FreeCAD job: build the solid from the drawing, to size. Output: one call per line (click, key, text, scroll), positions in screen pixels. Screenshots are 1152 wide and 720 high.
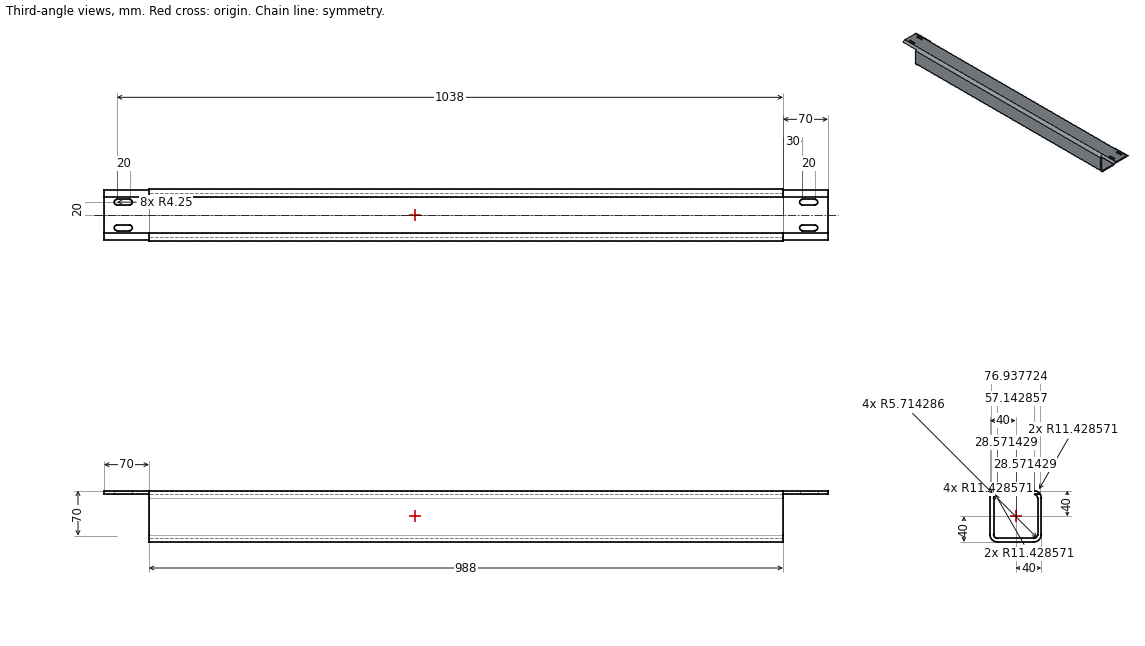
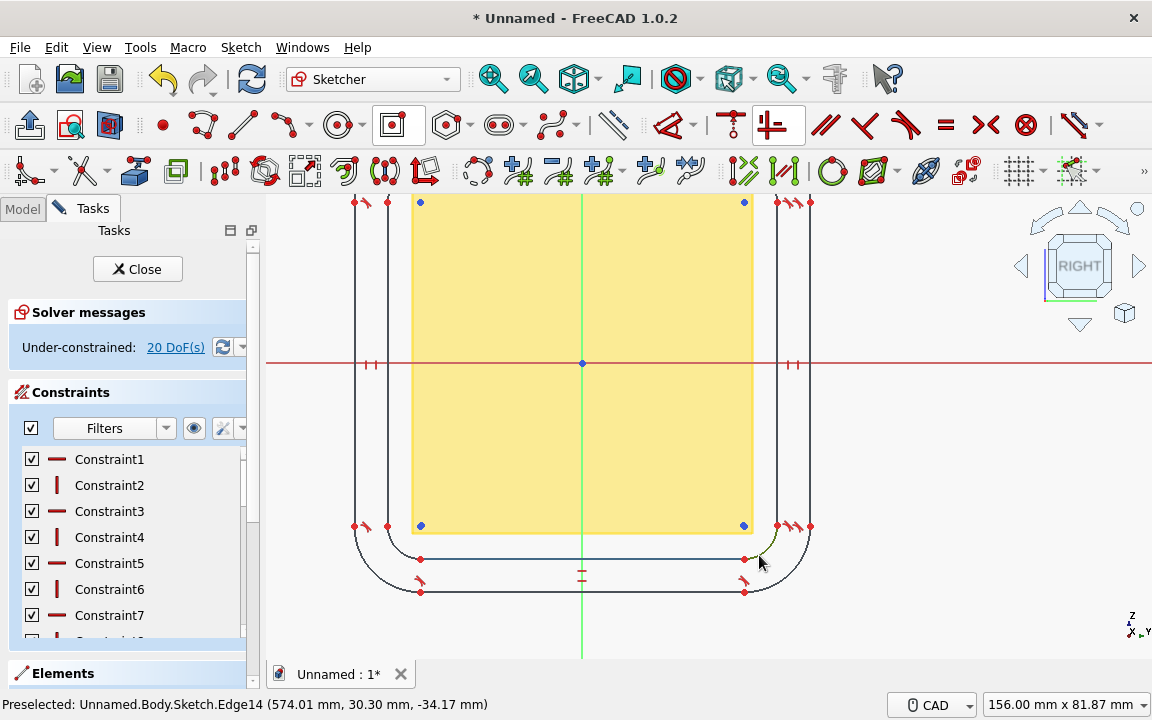
key(t)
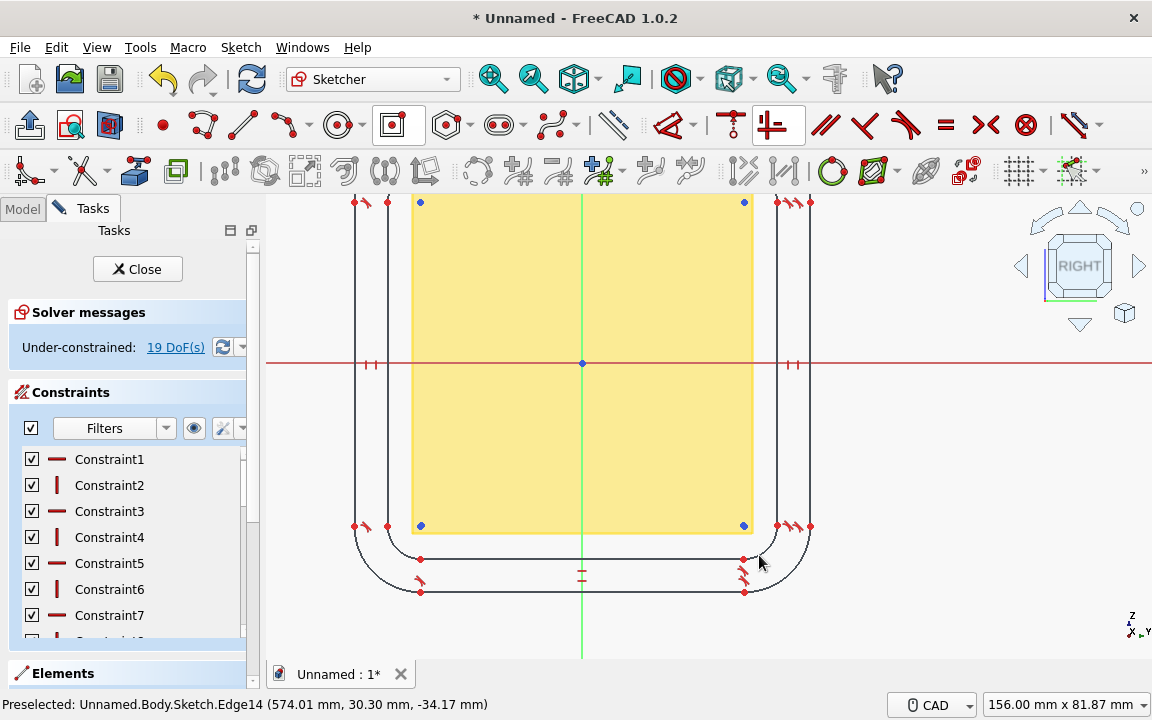
click(647, 559)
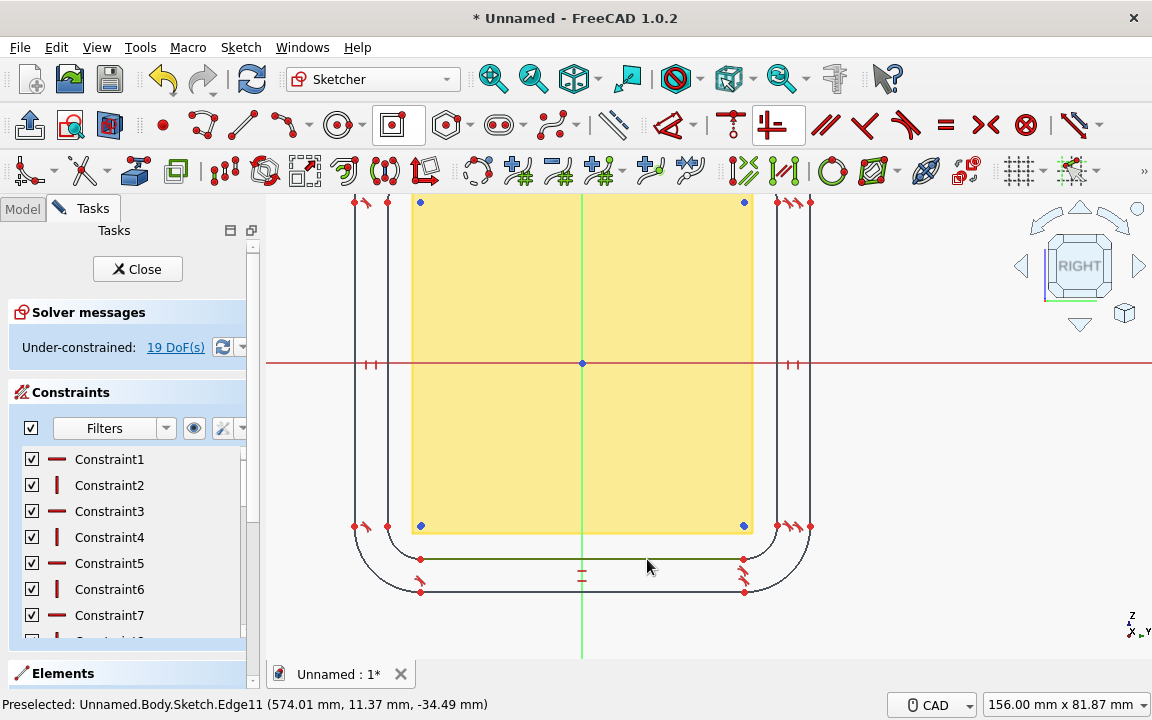
click(391, 541)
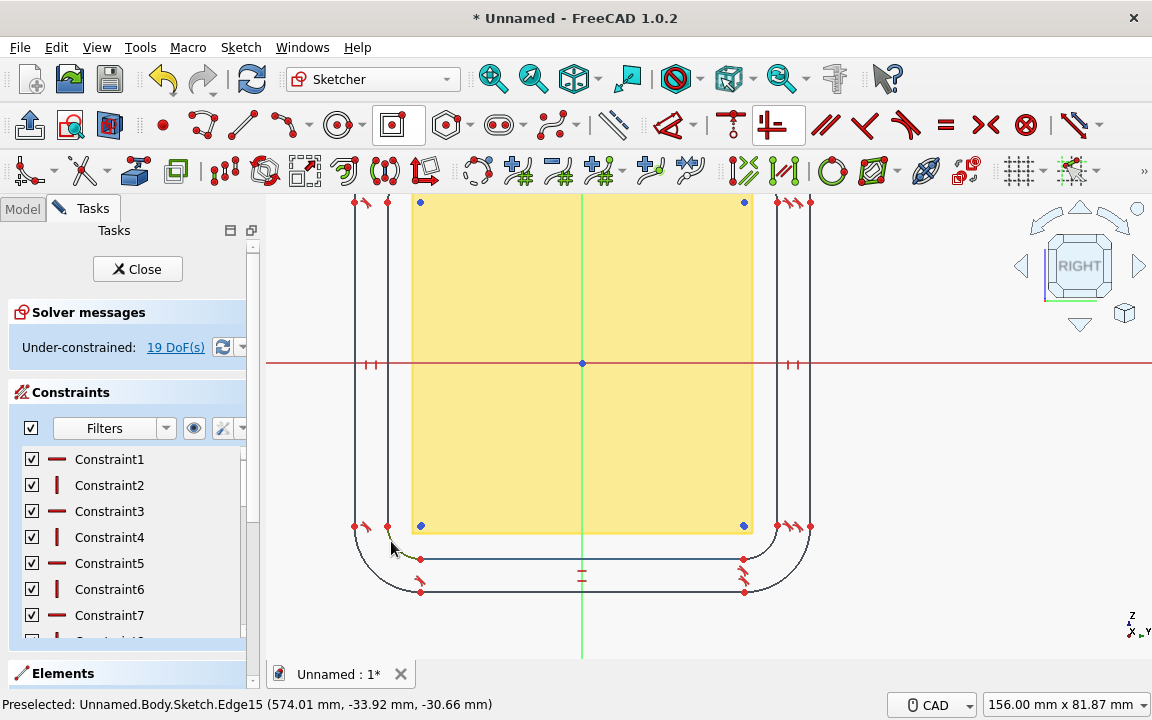
key(t)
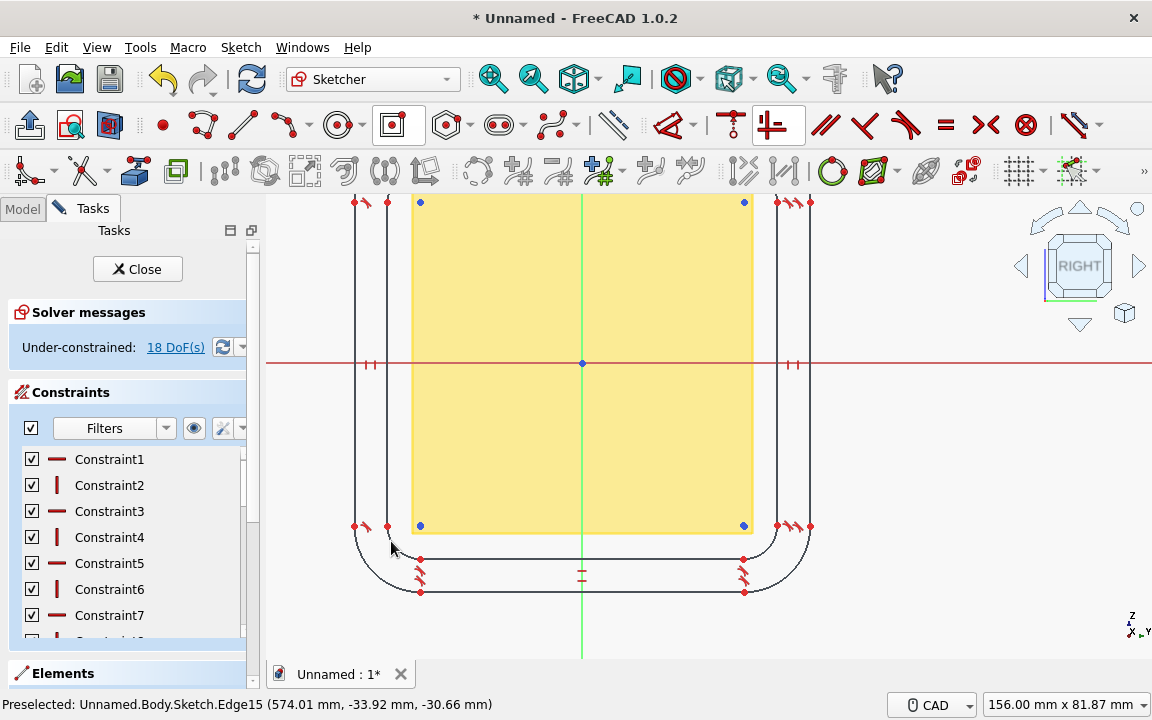
click(387, 429)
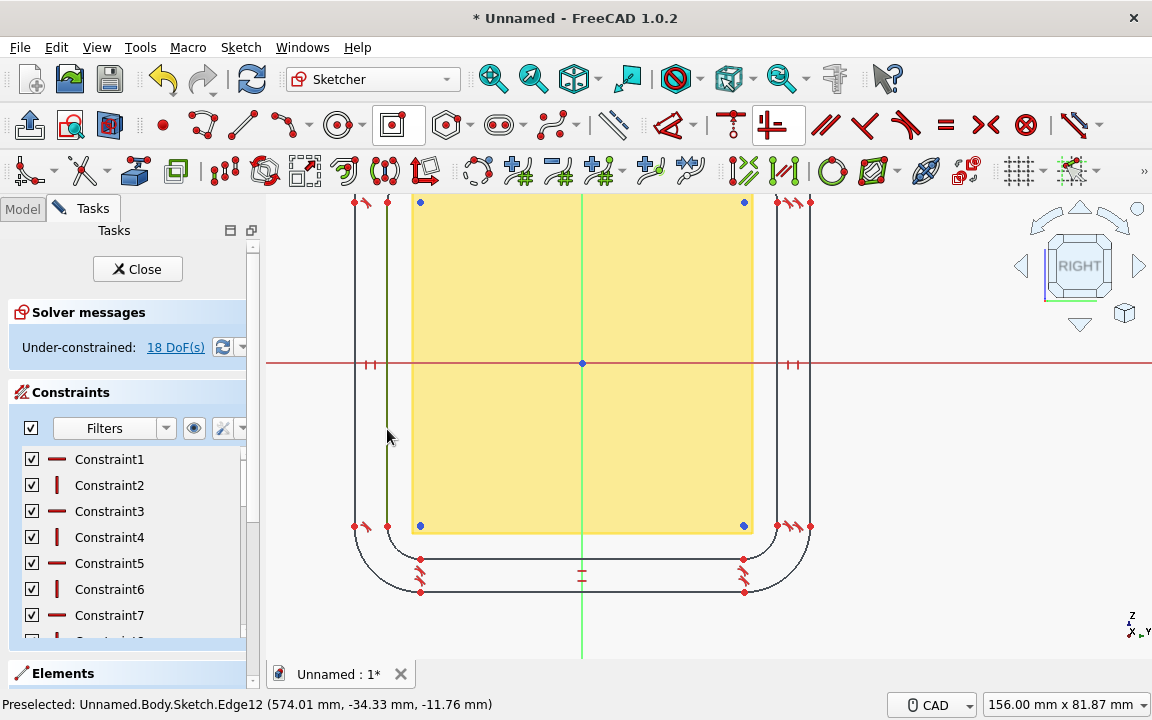
click(391, 541)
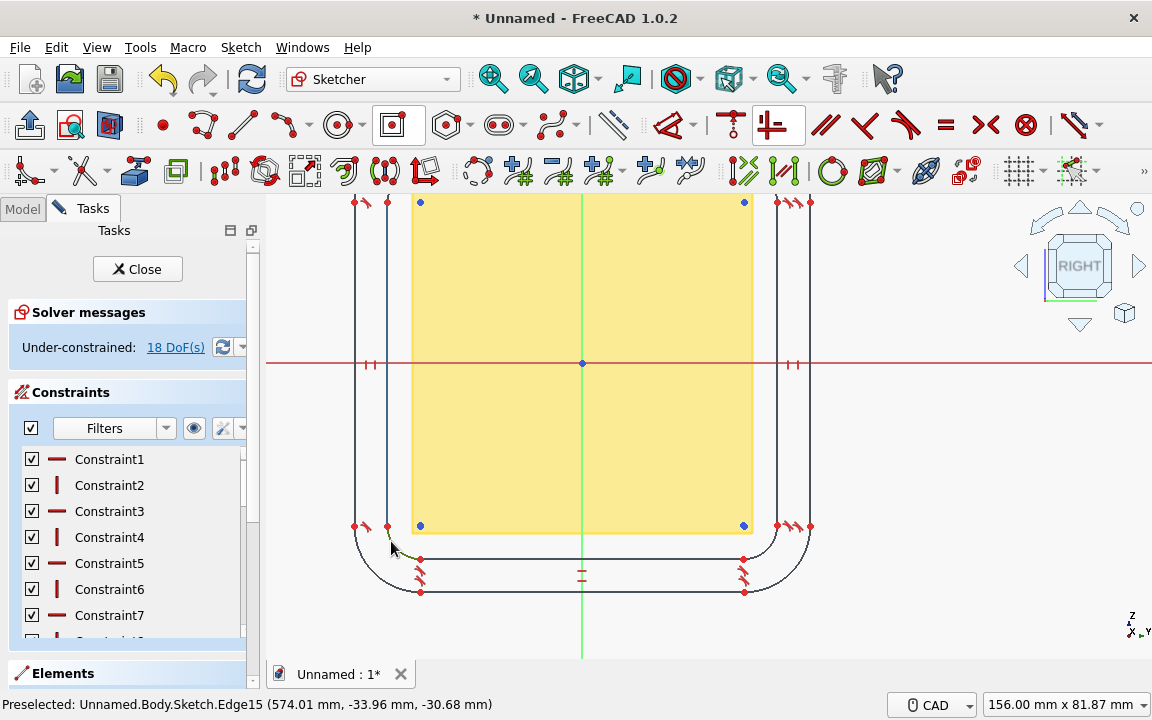
click(906, 126)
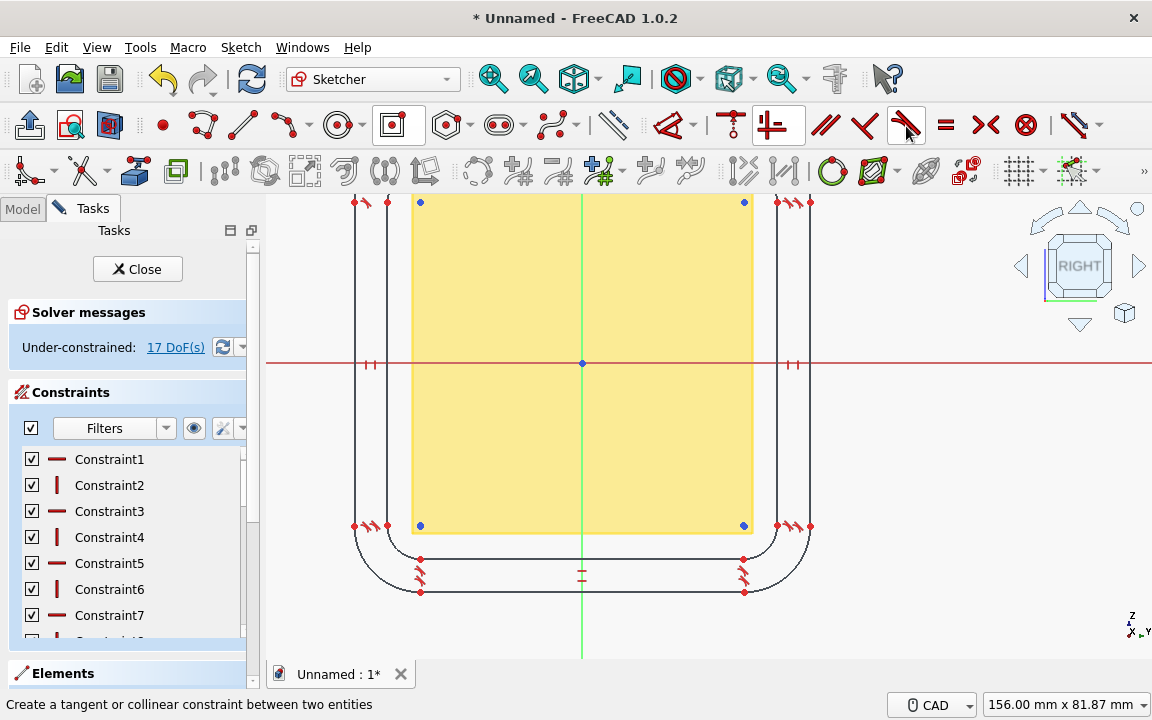
click(387, 429)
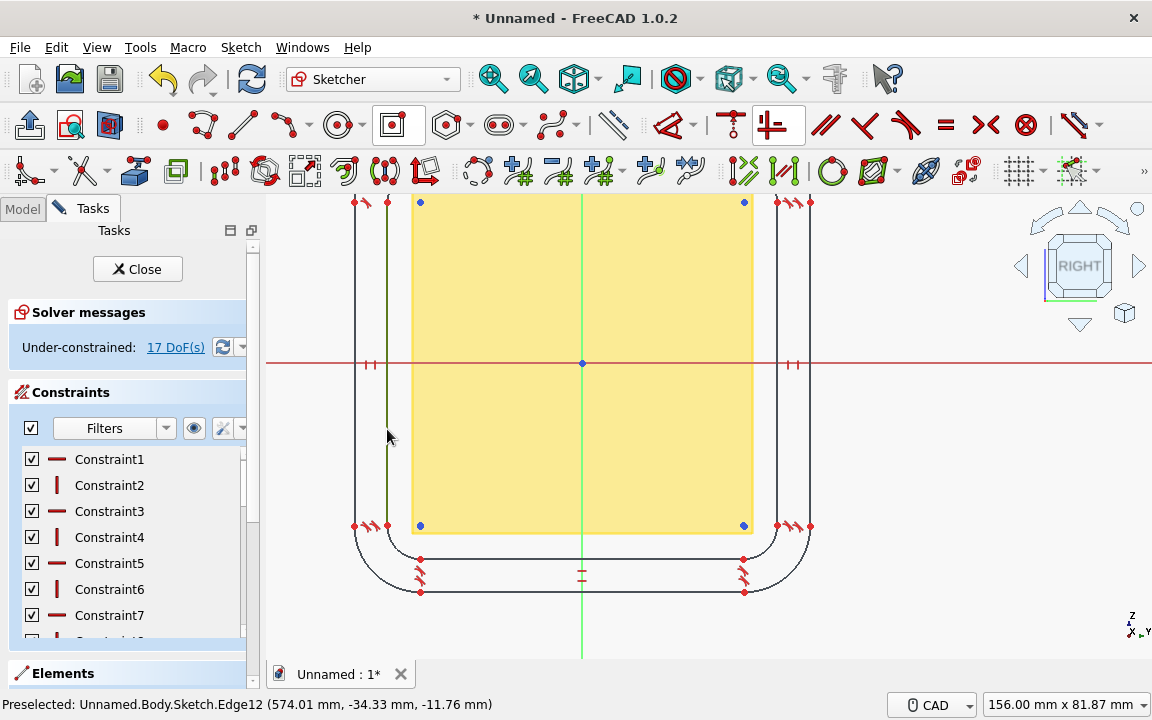
scroll(759, 555, down, 2)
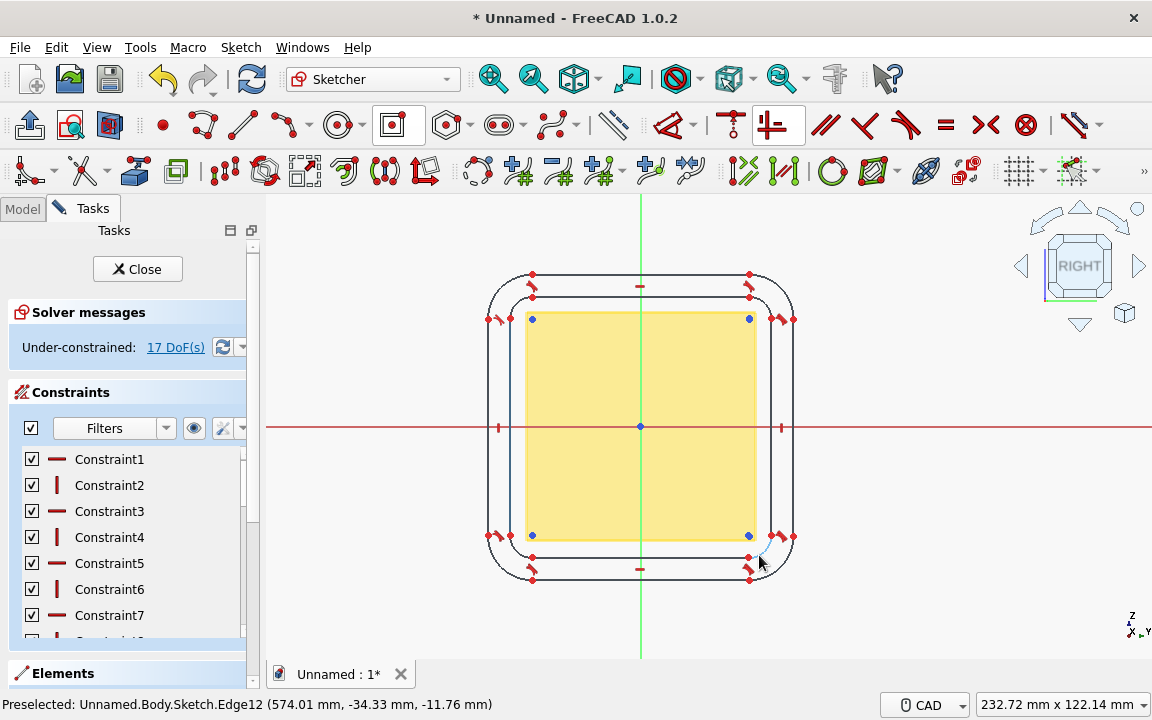
scroll(522, 299, up, 2)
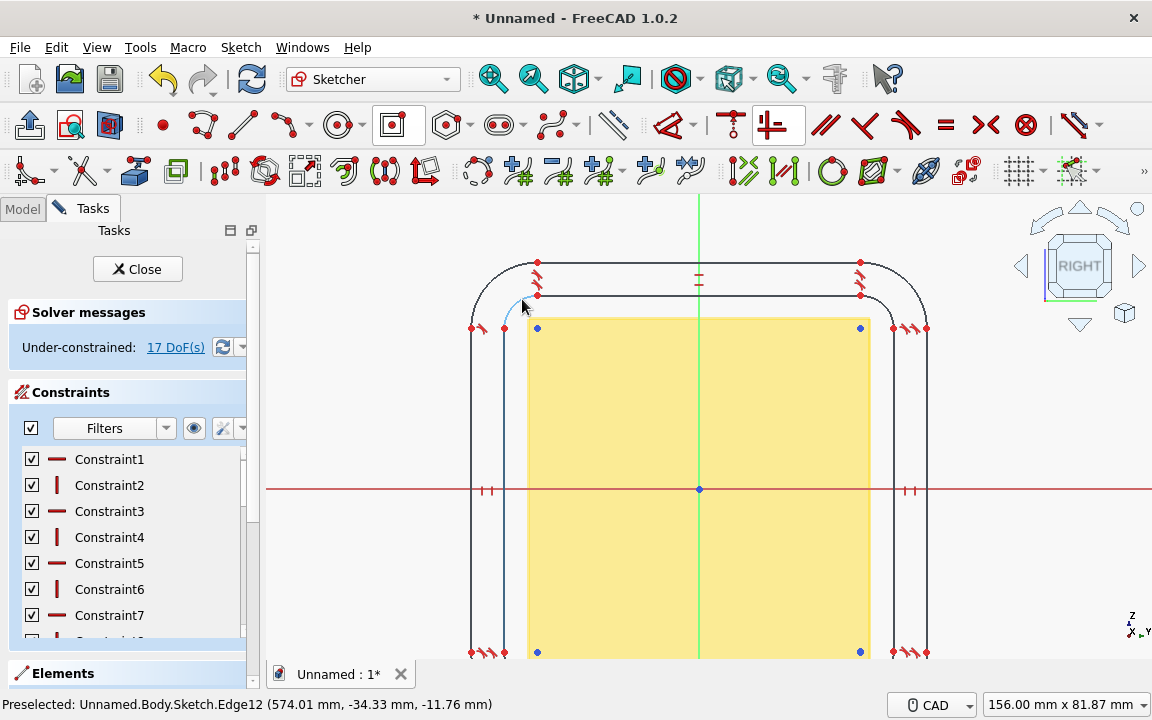
click(522, 299)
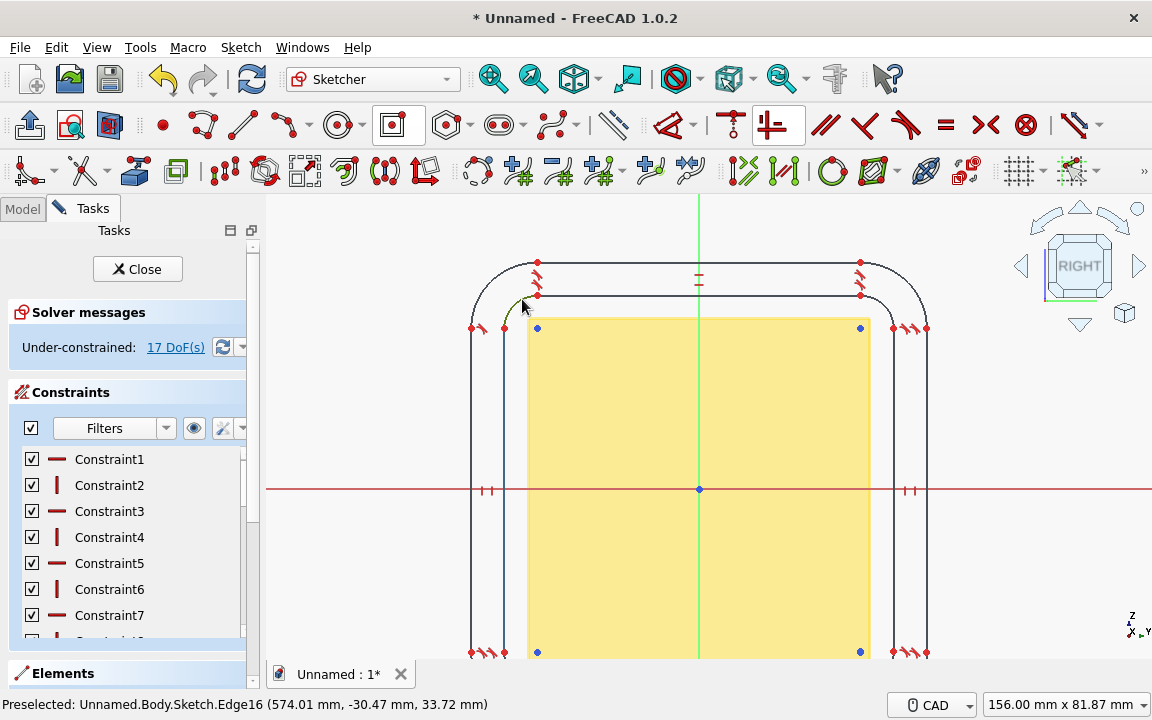
key(t)